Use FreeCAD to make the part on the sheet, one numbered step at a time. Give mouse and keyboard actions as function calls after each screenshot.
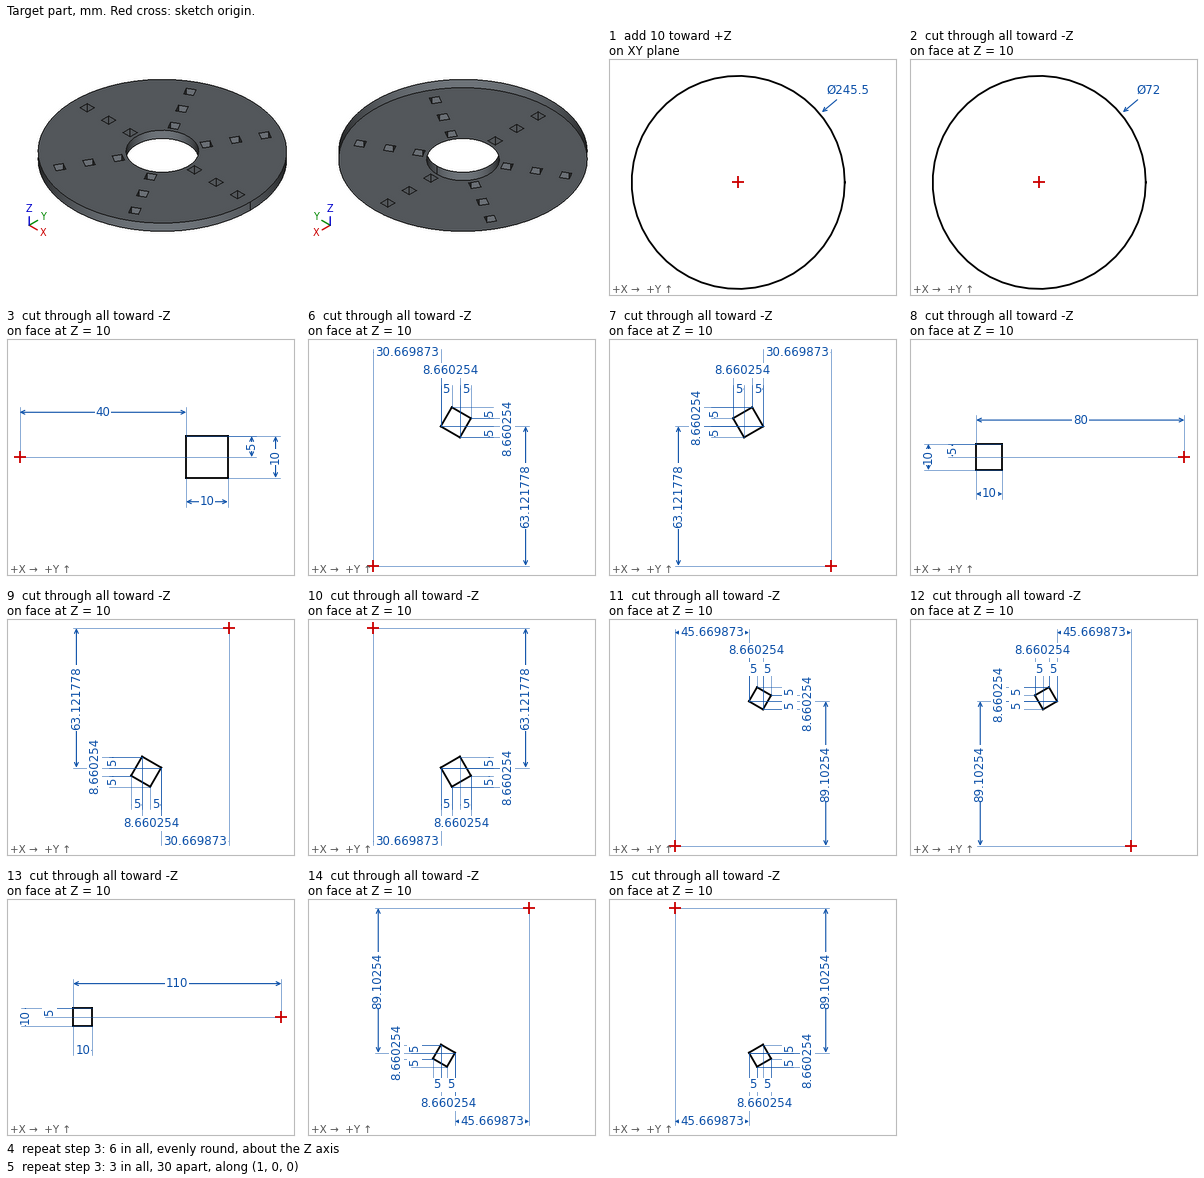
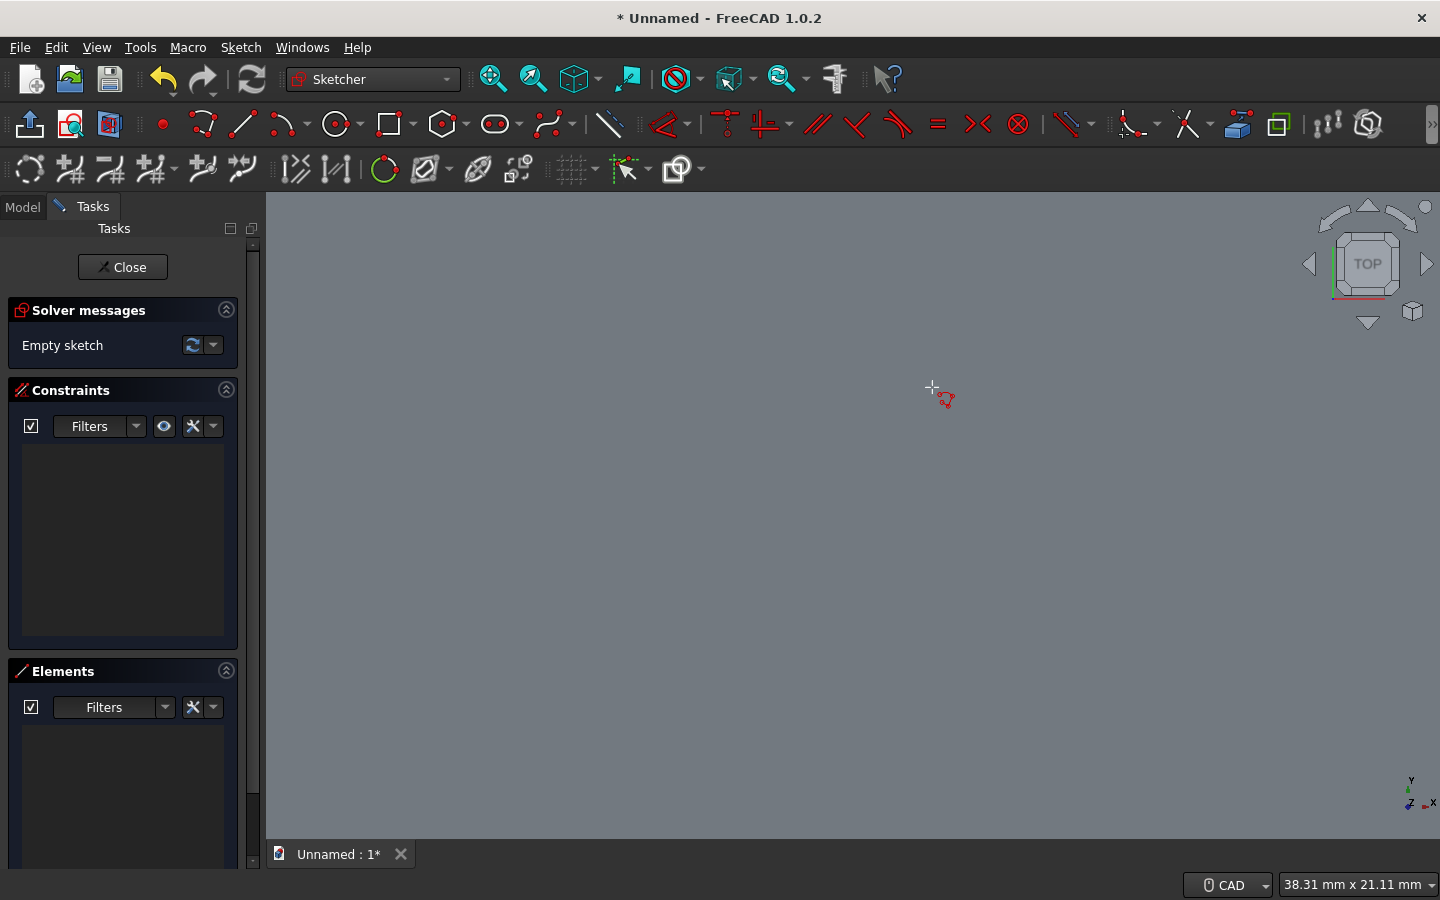
click(562, 561)
click(827, 714)
click(980, 449)
click(715, 296)
click(562, 562)
key(Escape)
key(Escape)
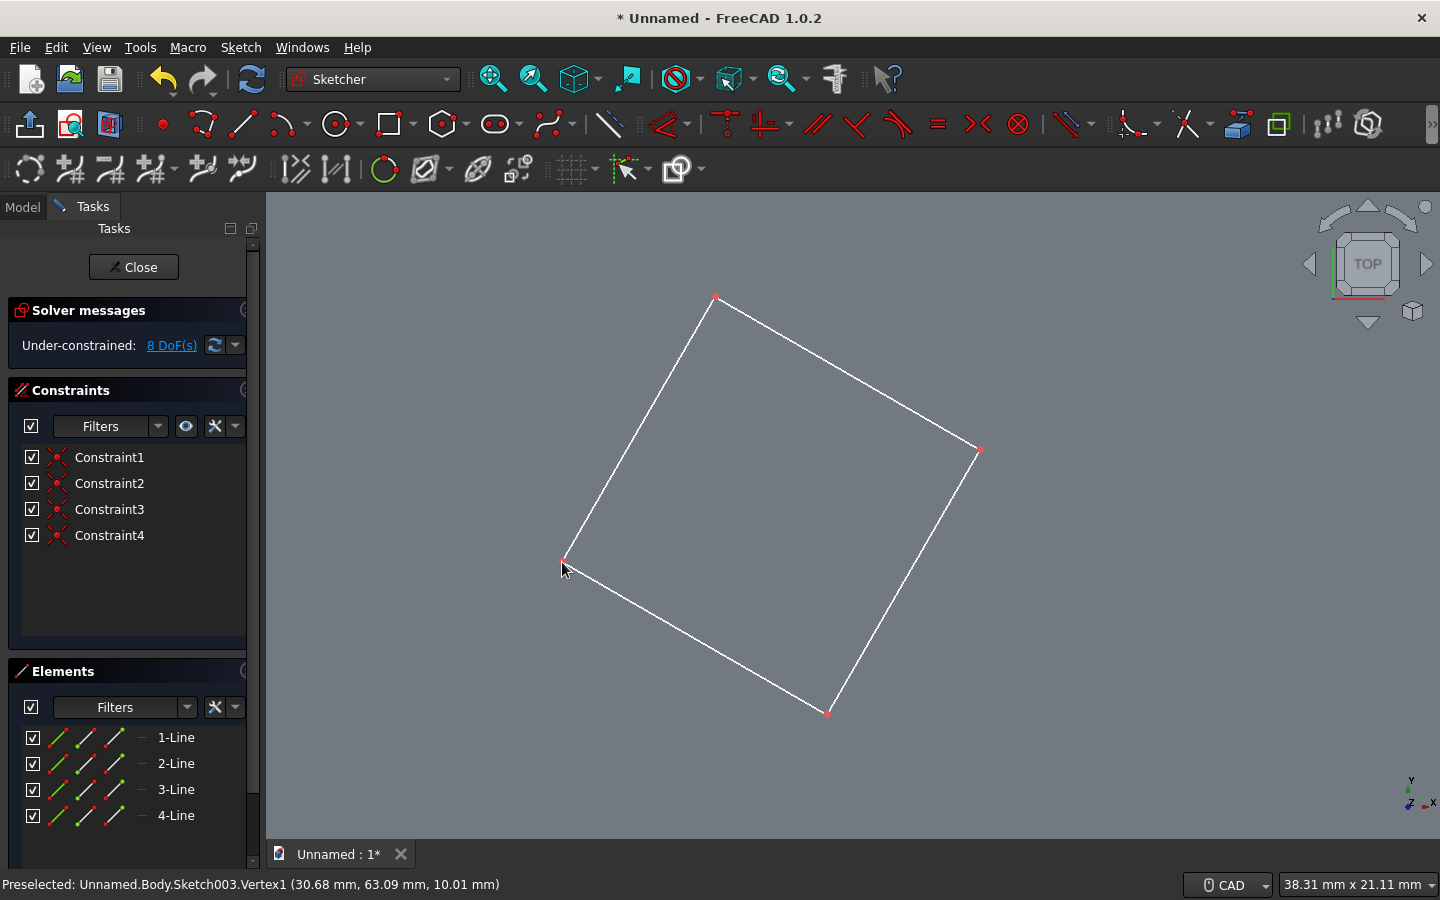
key(d)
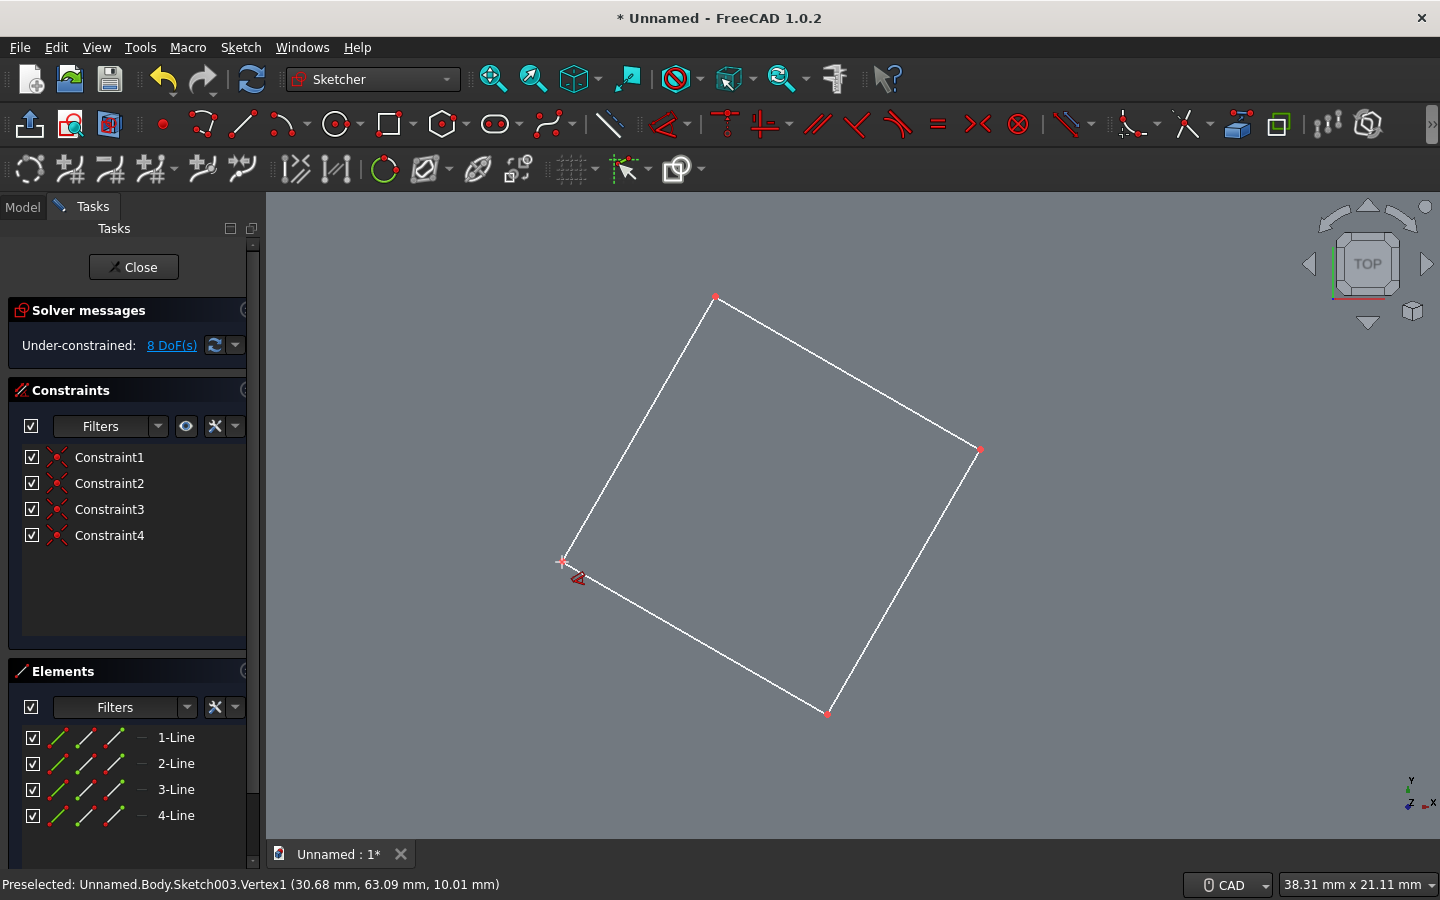
click(642, 608)
click(528, 639)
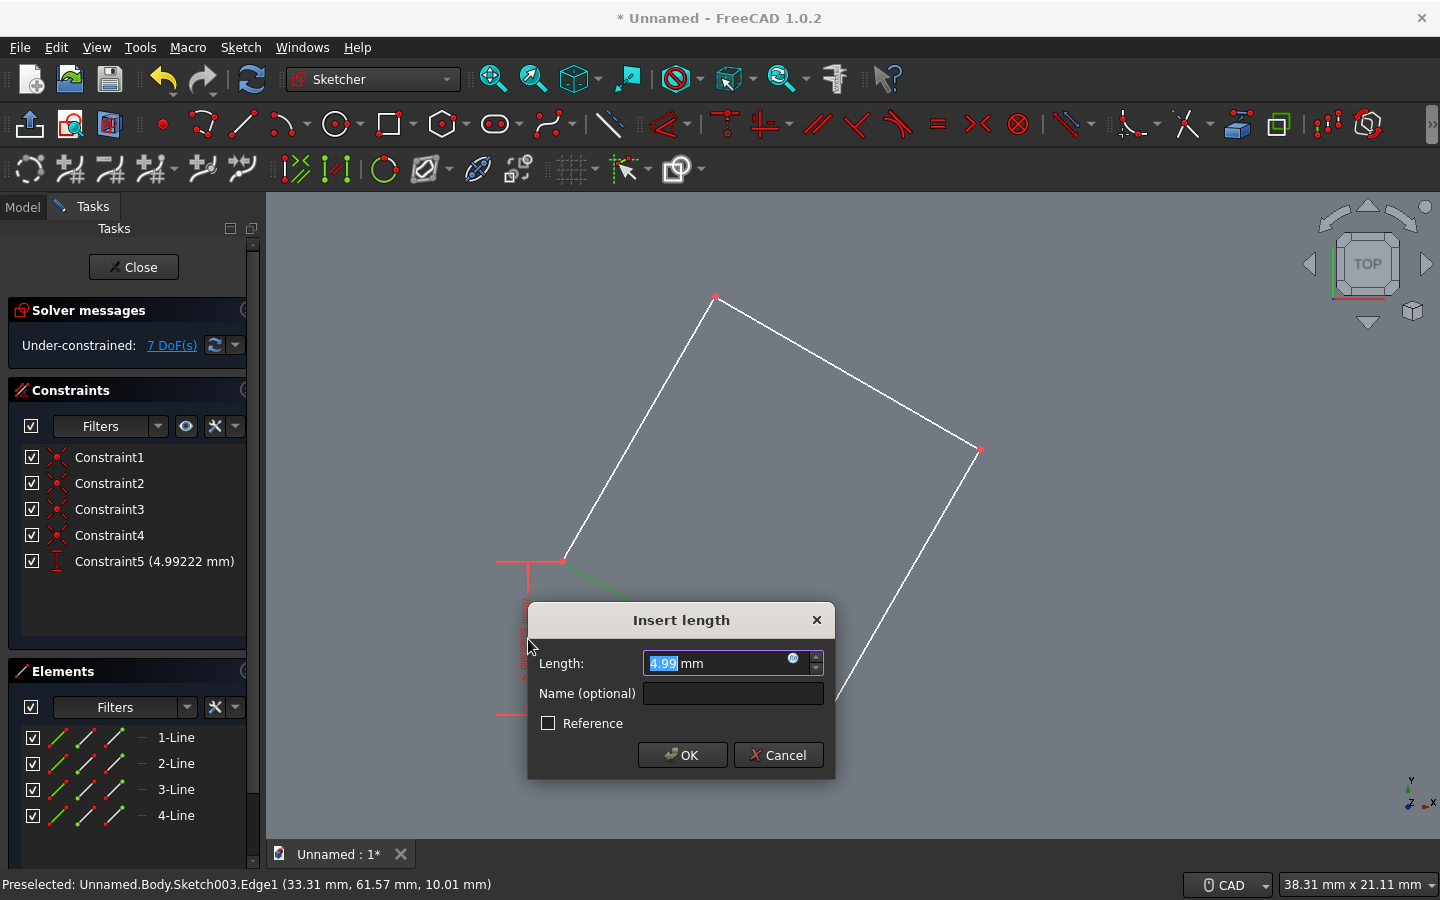
text(5)
key(Return)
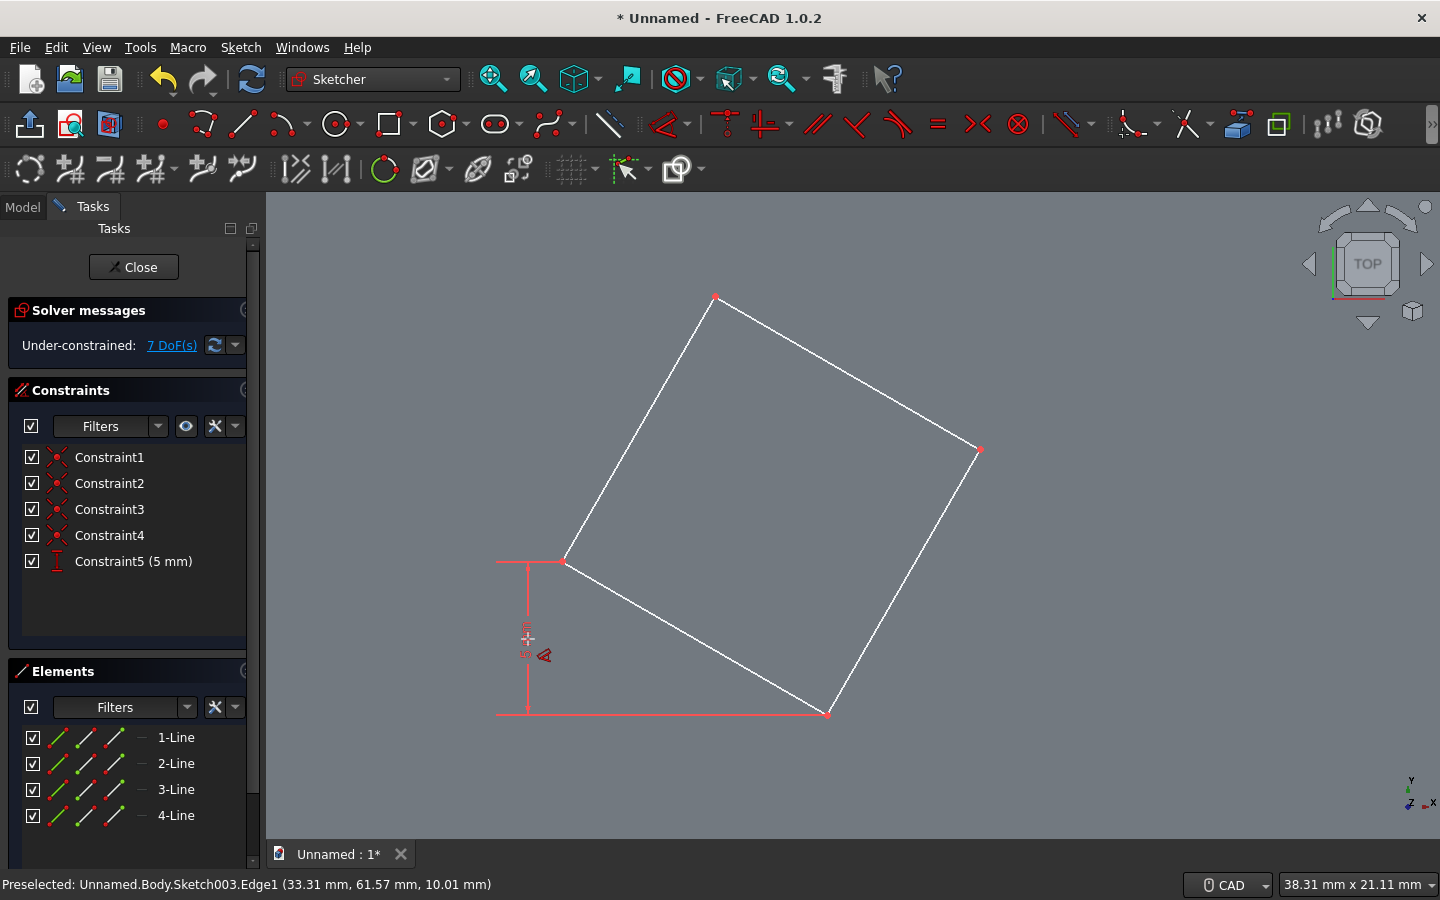
click(873, 636)
click(904, 749)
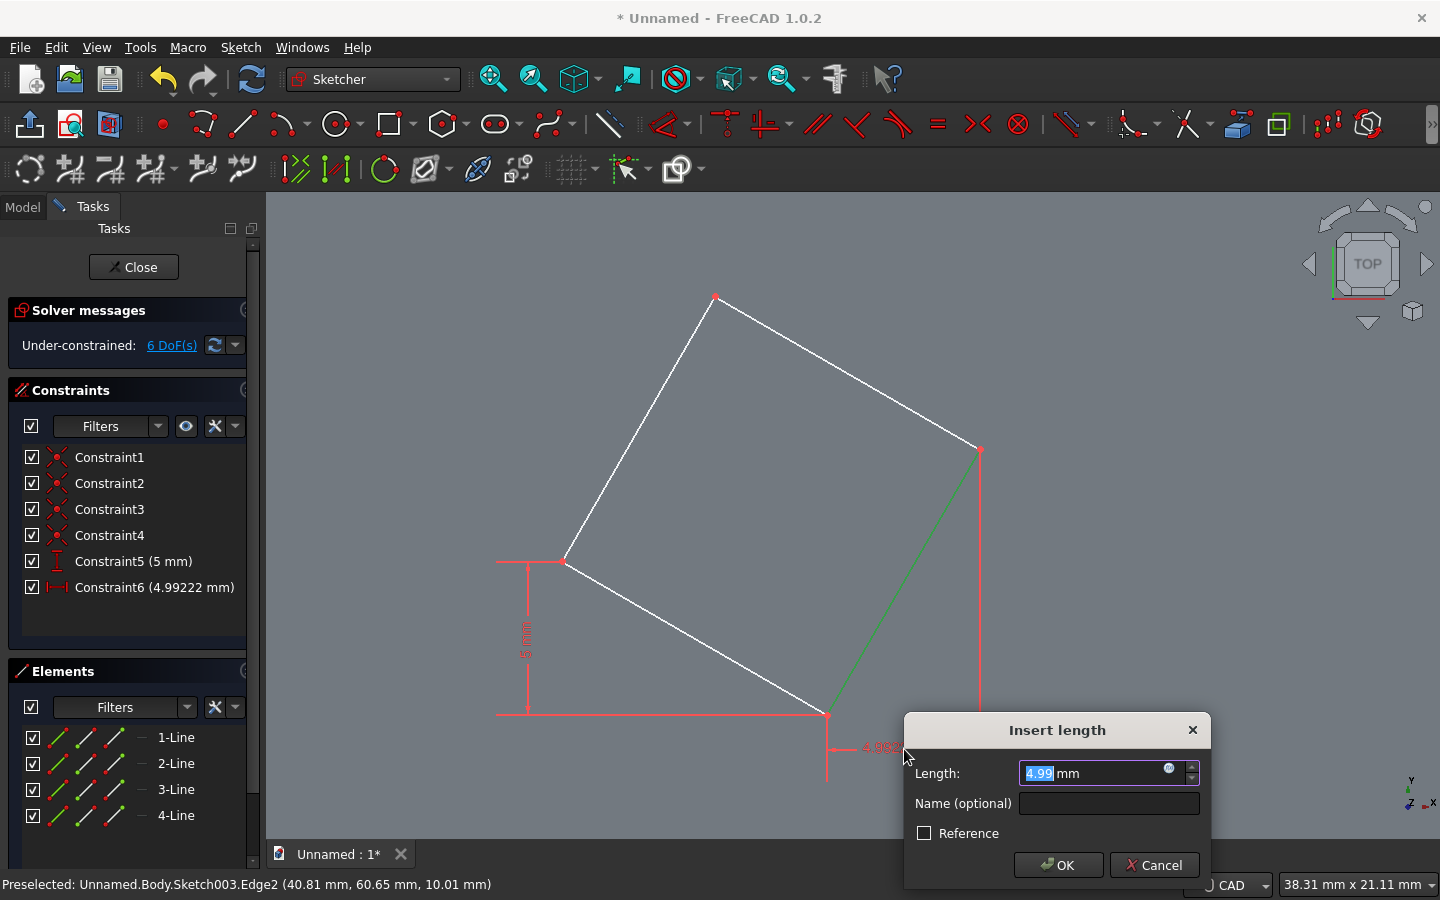
text(5)
key(Return)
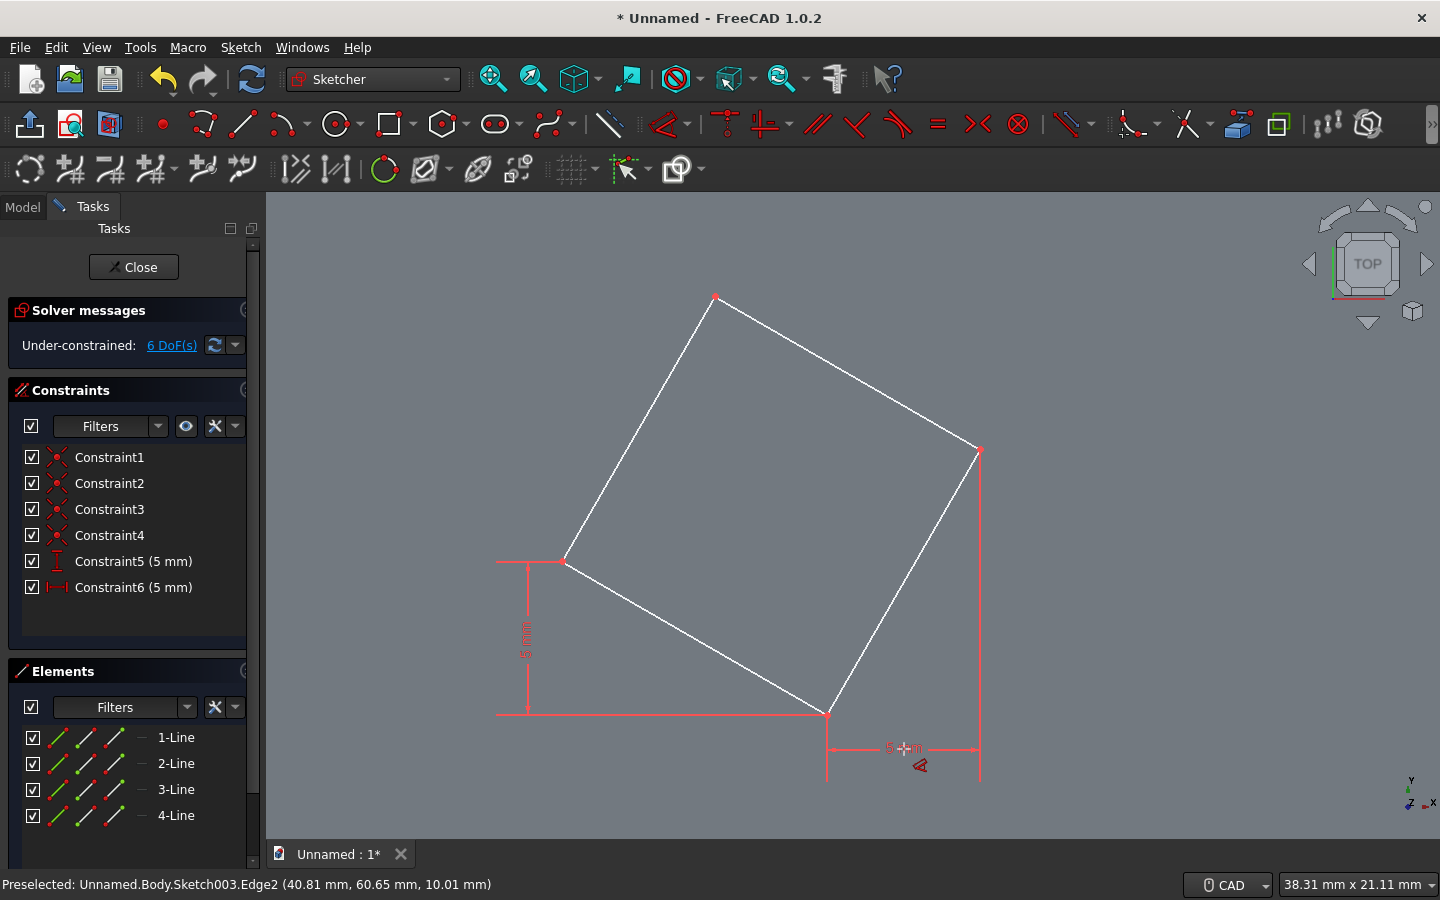
click(901, 404)
click(1014, 373)